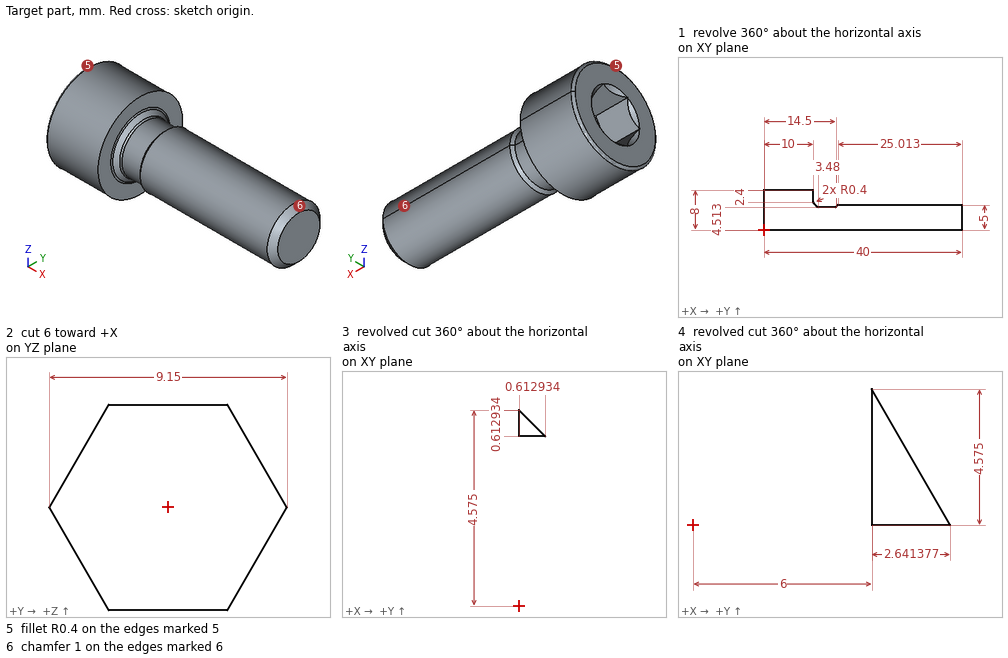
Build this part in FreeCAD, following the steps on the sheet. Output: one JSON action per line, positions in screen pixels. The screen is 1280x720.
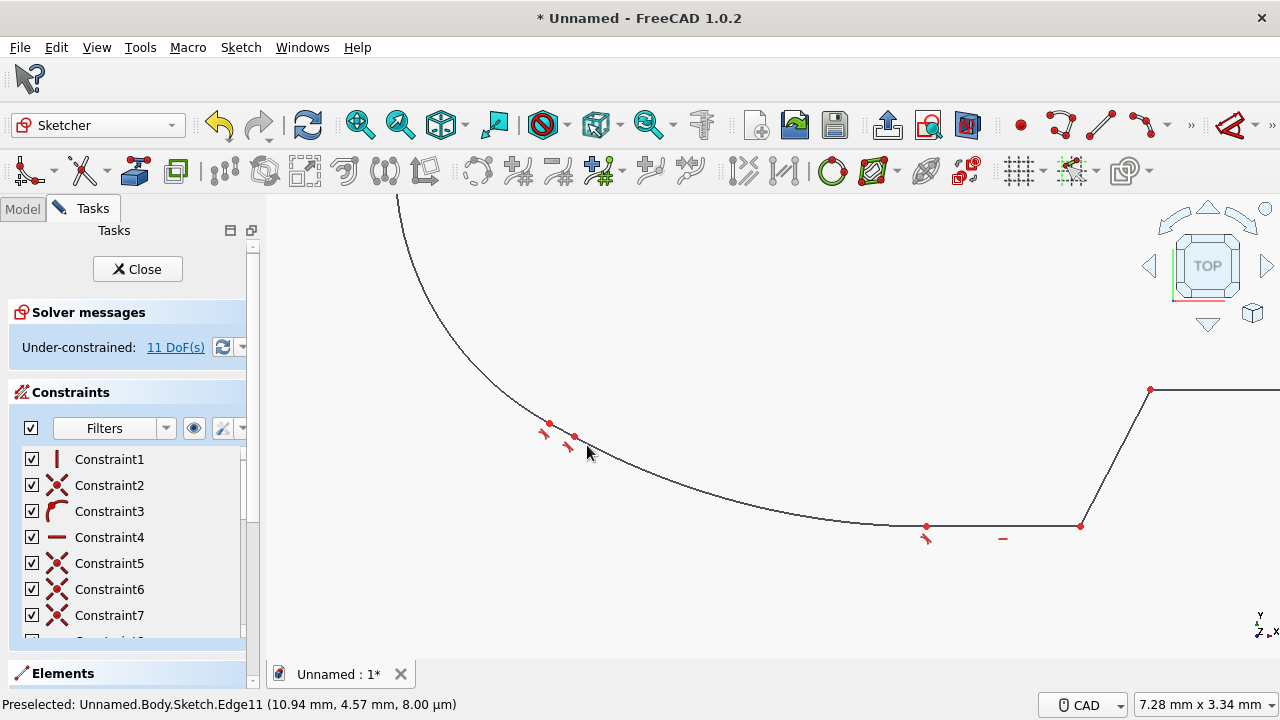
{"action": "scroll", "coordinate": [562, 415], "scroll_direction": "down", "scroll_amount": 11}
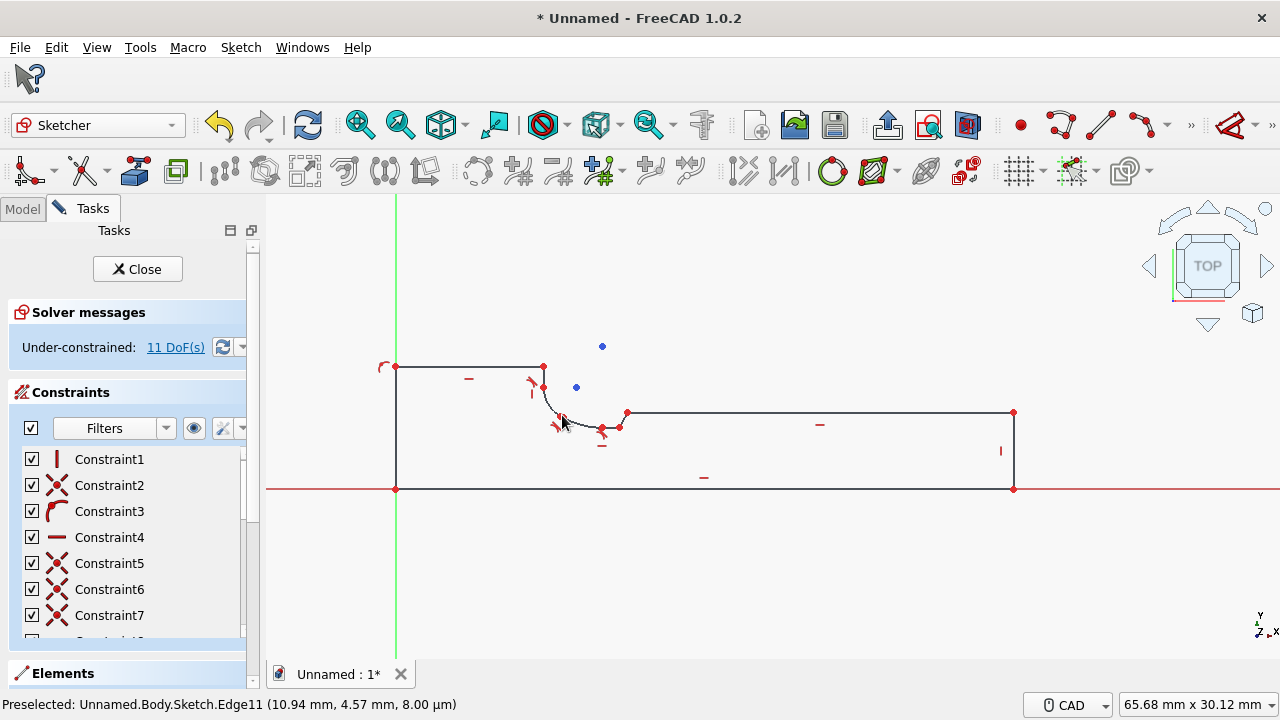
{"action": "scroll", "coordinate": [545, 398], "scroll_direction": "up", "scroll_amount": 2}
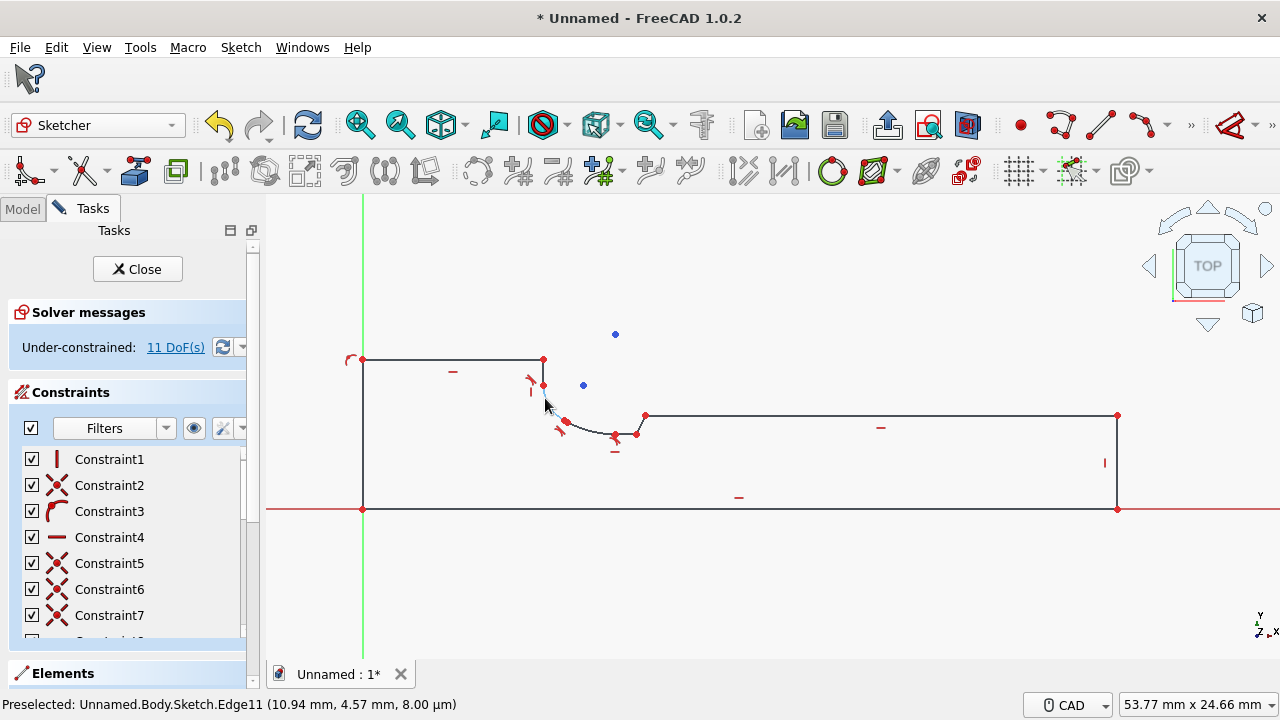
{"action": "left_click", "coordinate": [546, 398]}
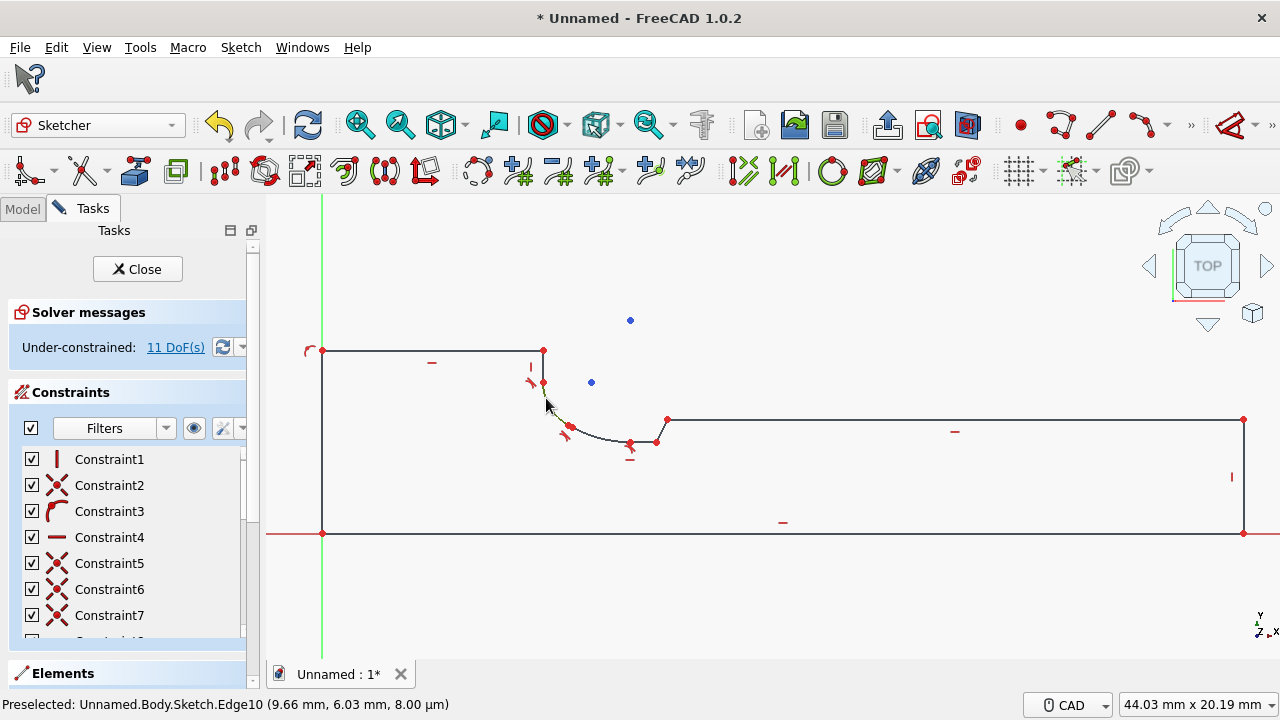
{"action": "left_click", "coordinate": [589, 435]}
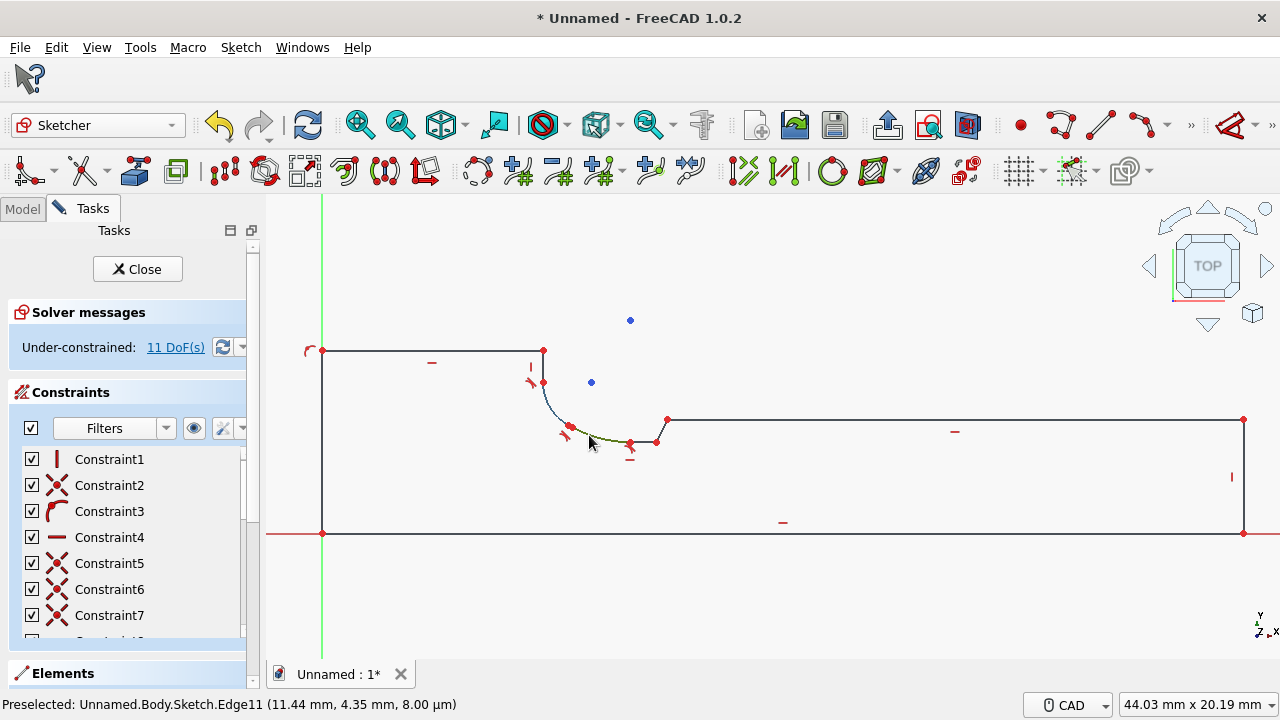
{"action": "key", "text": "e"}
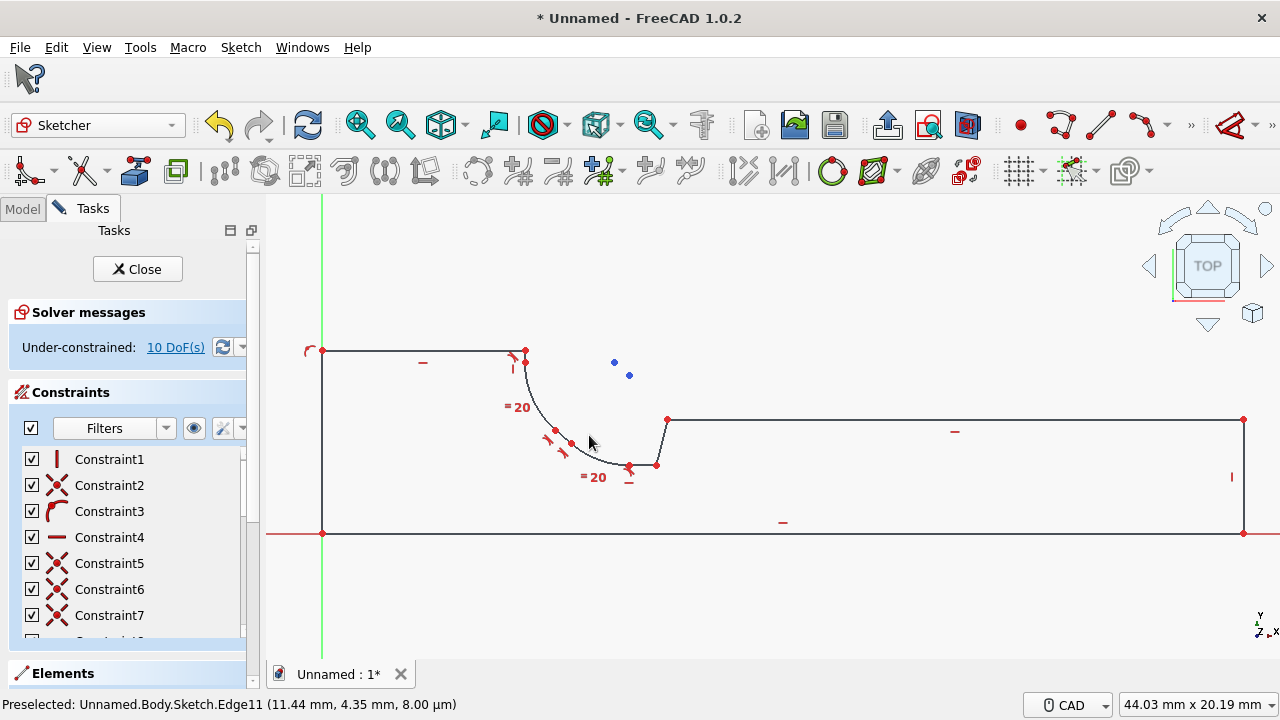
{"action": "scroll", "coordinate": [528, 385], "scroll_direction": "up", "scroll_amount": 8}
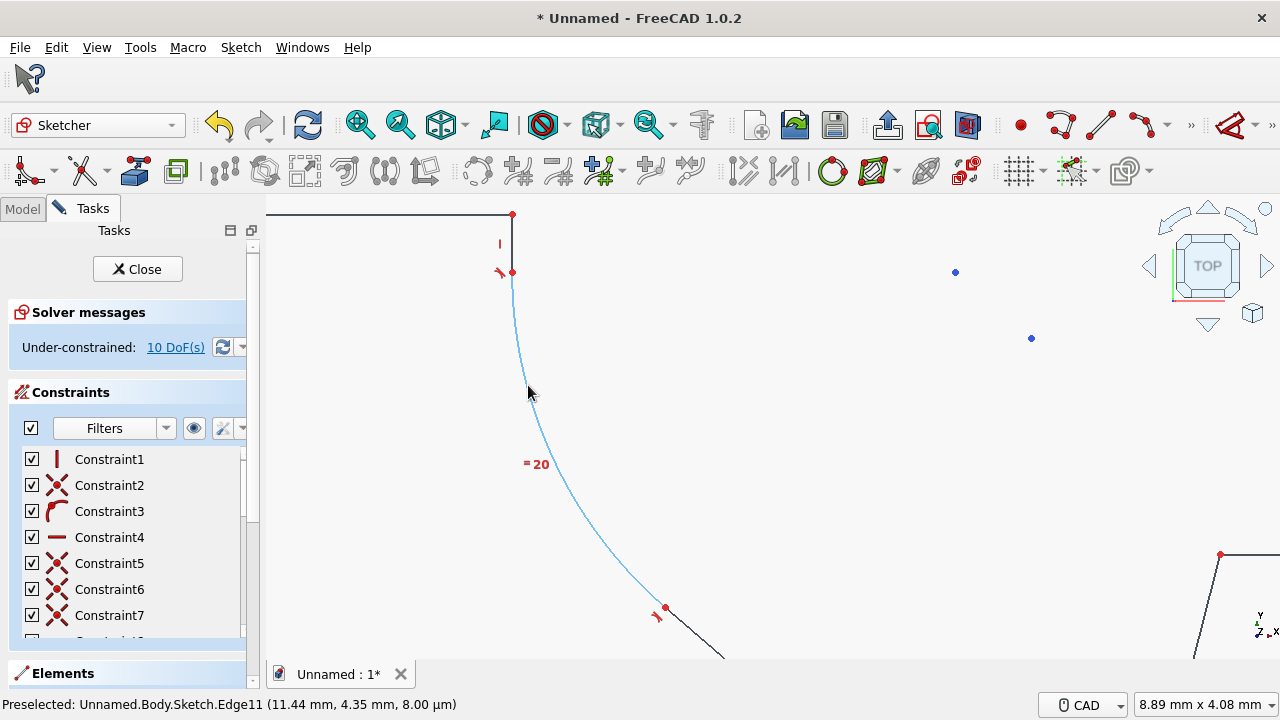
{"action": "left_click", "coordinate": [527, 385]}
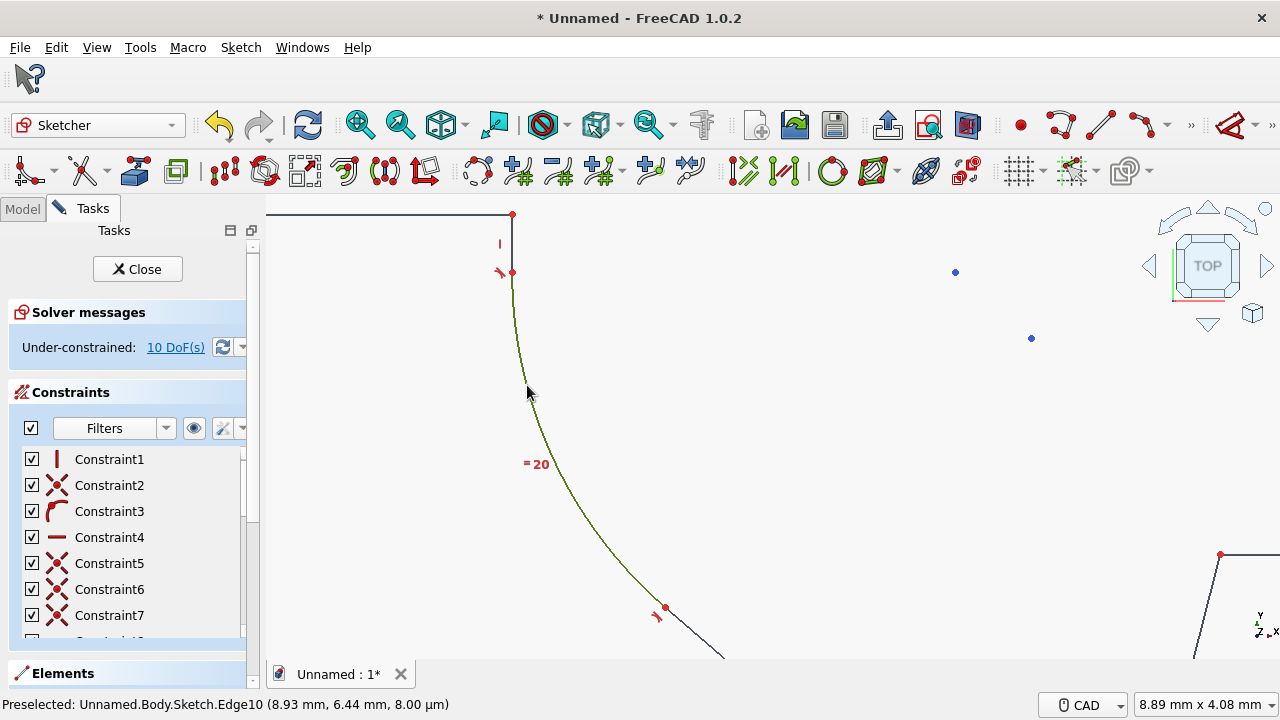
{"action": "left_click", "coordinate": [1258, 126]}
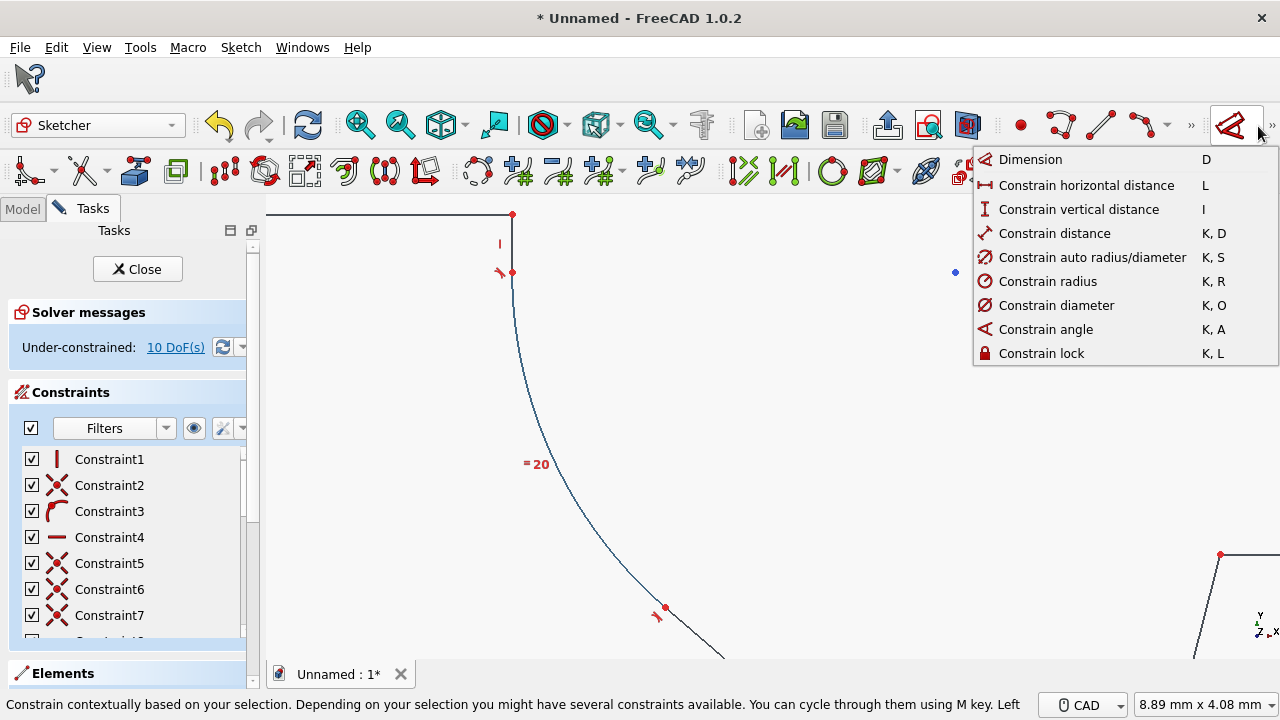
{"action": "left_click", "coordinate": [1126, 281]}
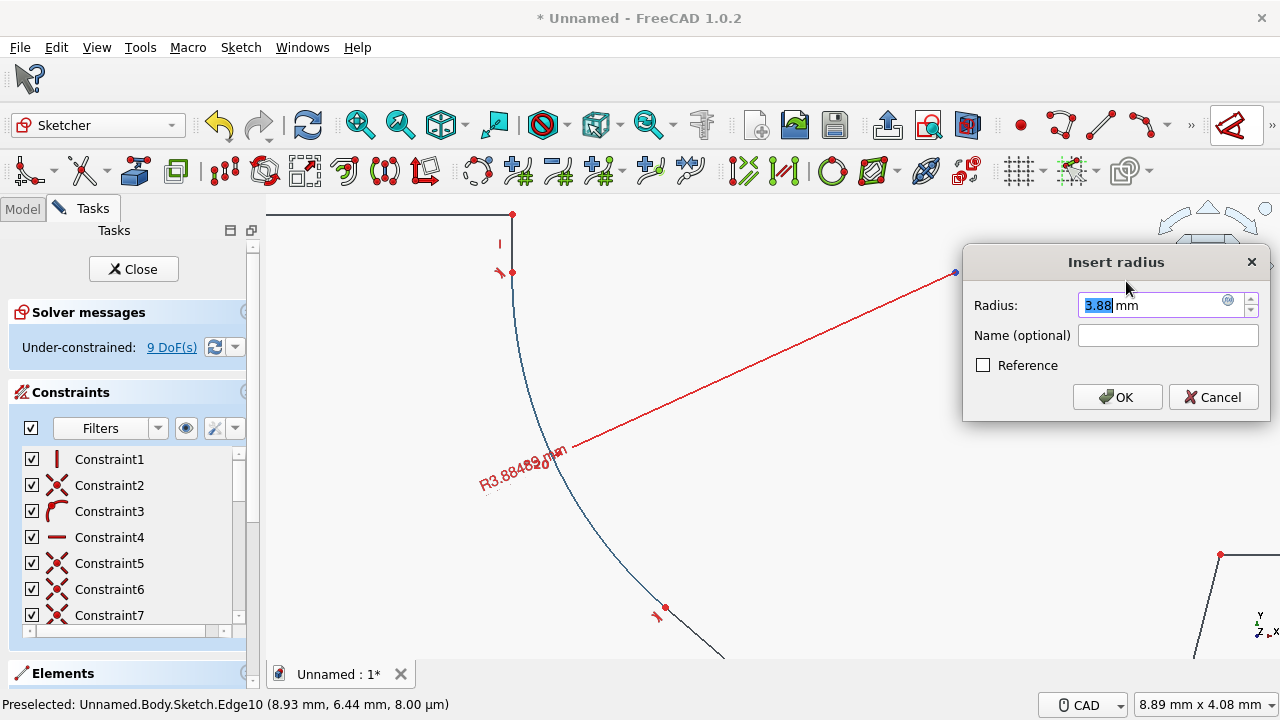
{"action": "type", "text": "0.4"}
{"action": "key", "text": "Return"}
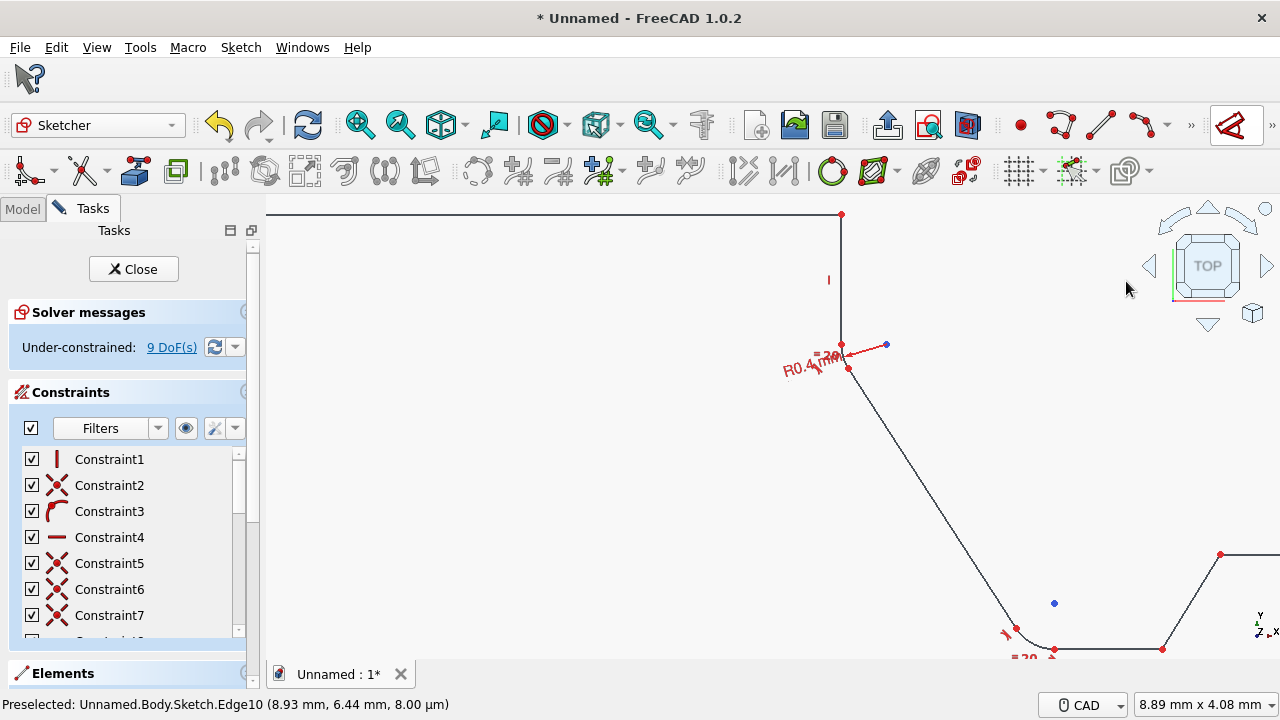
{"action": "scroll", "coordinate": [535, 389], "scroll_direction": "down", "scroll_amount": 10}